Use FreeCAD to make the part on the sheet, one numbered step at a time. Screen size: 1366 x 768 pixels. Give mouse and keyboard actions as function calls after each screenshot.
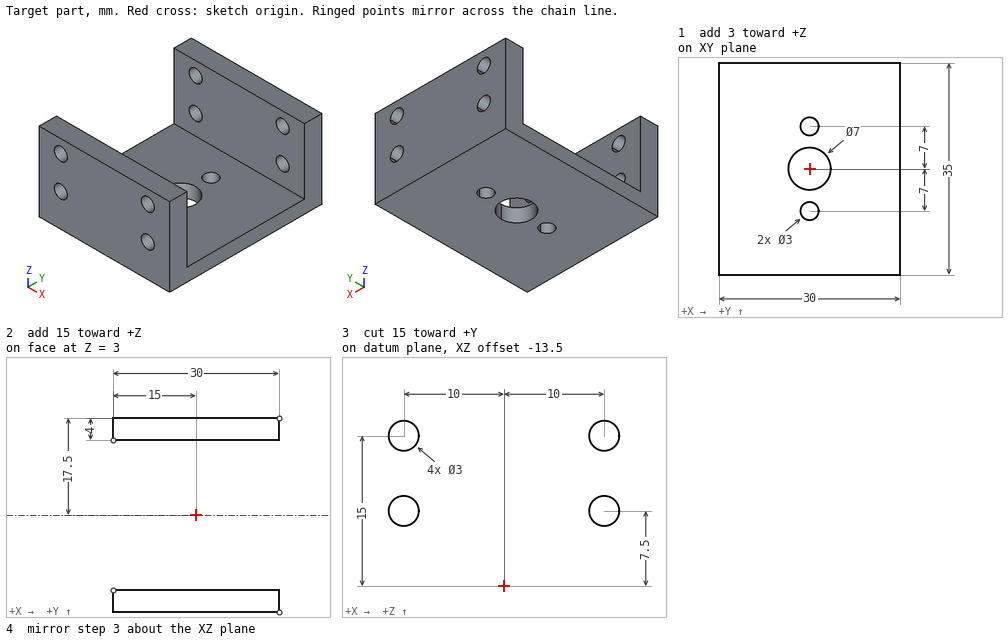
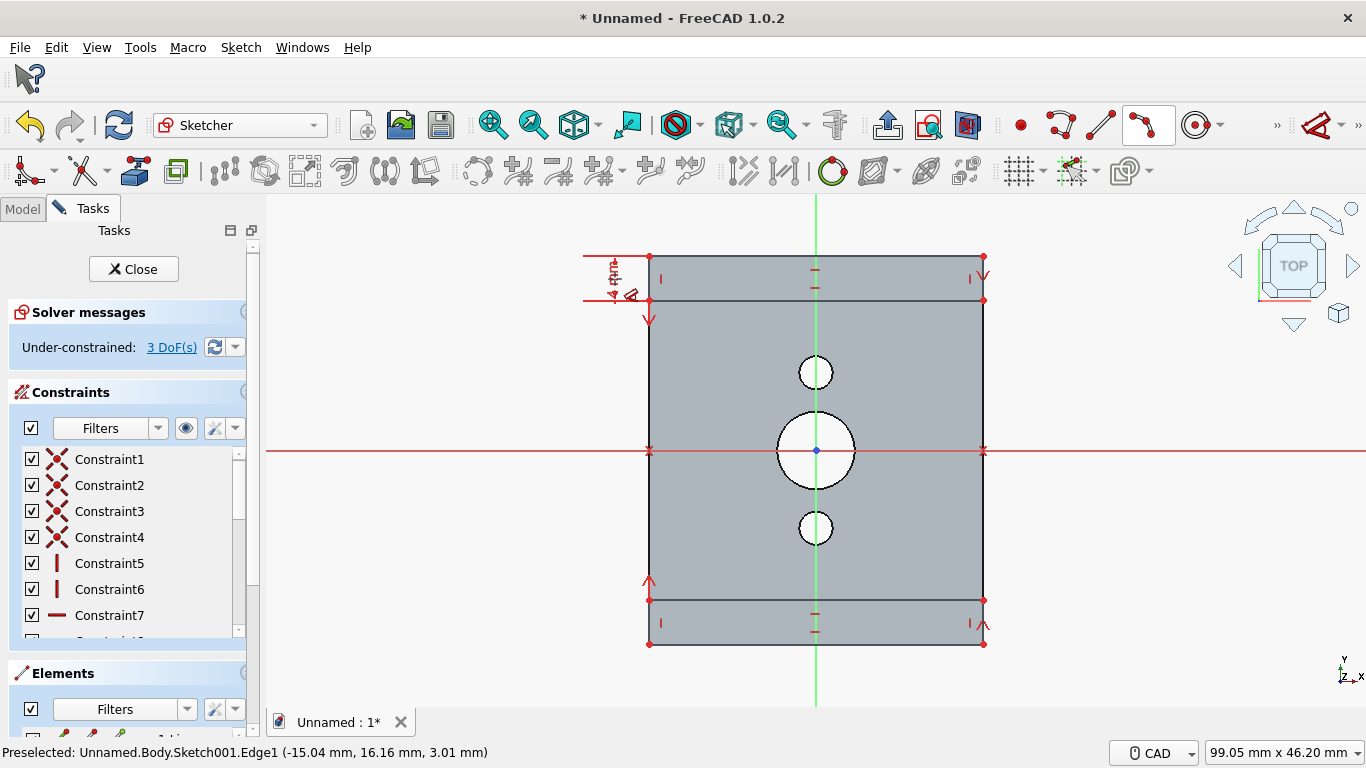
click(749, 301)
click(739, 335)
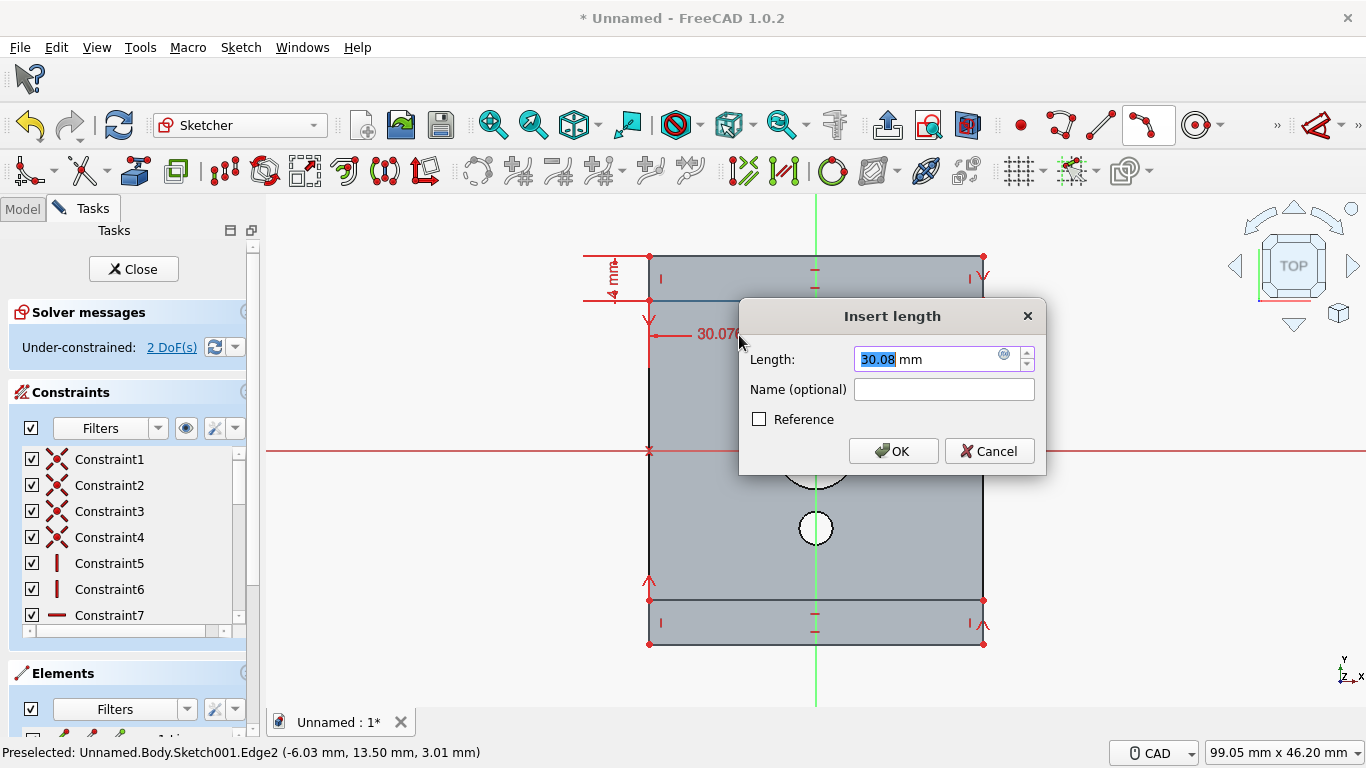
text(30)
key(Return)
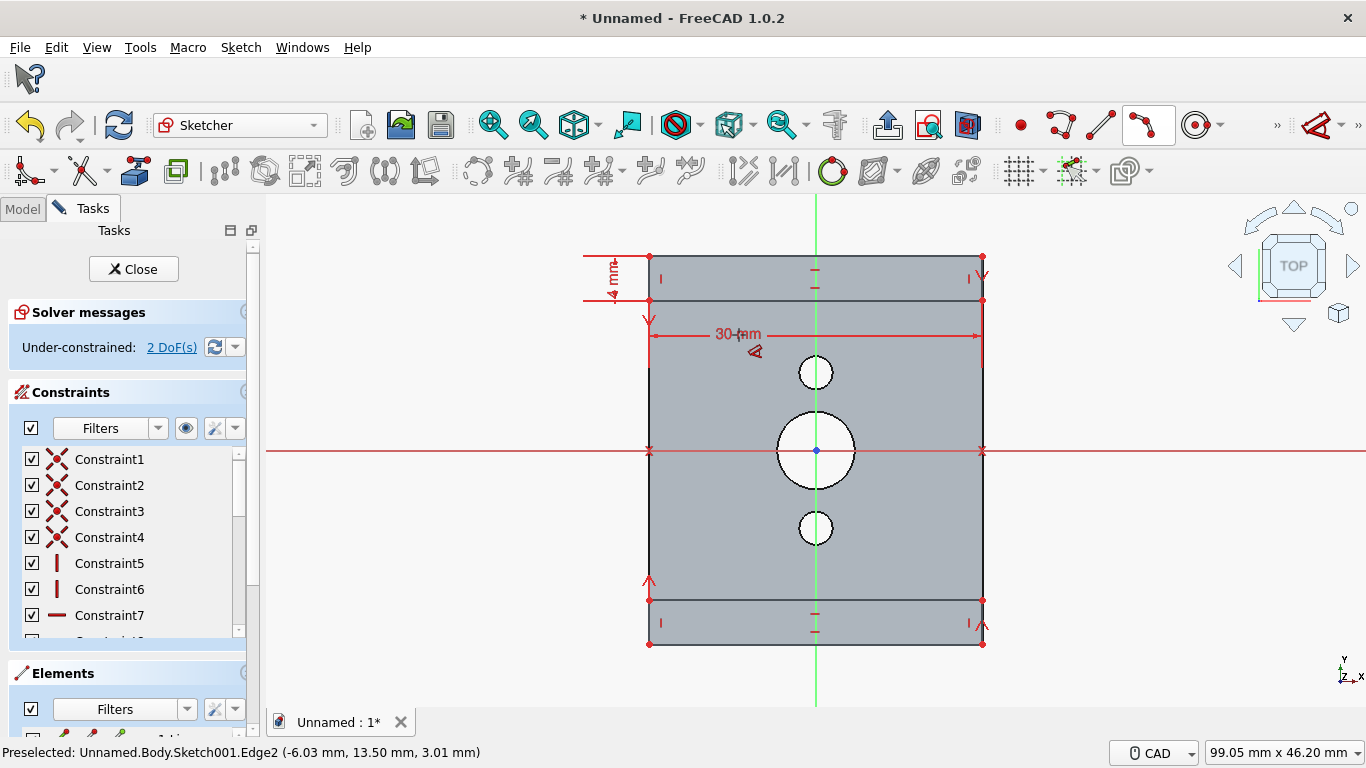
click(649, 256)
click(733, 222)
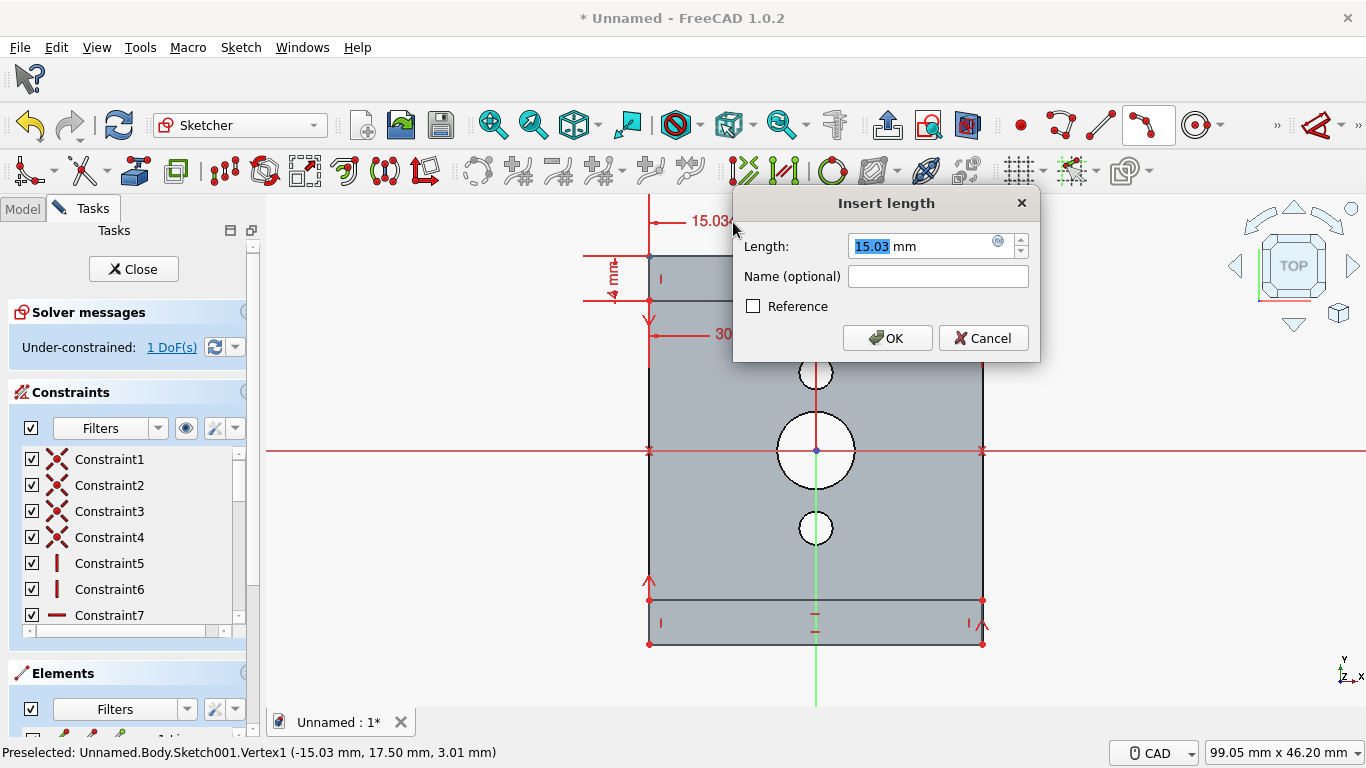
text(15)
key(Return)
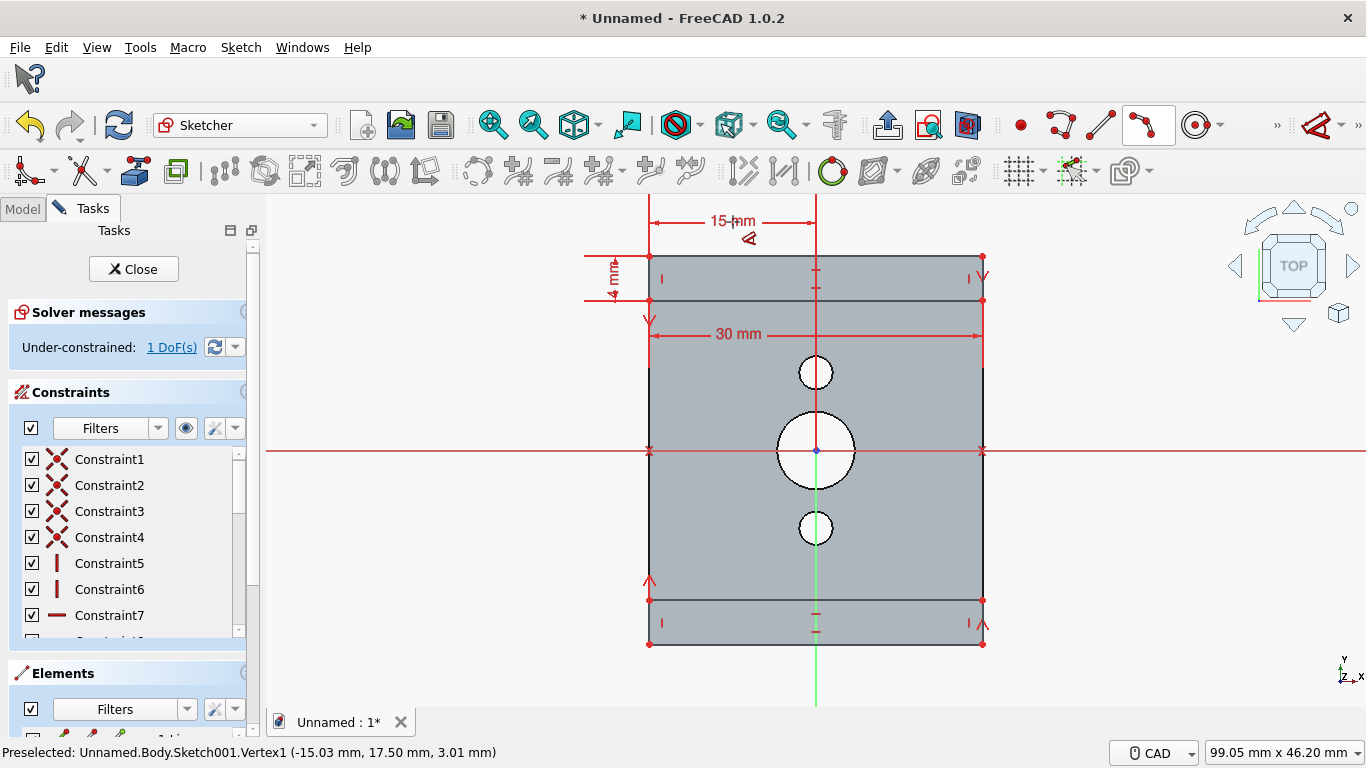
click(649, 256)
click(615, 353)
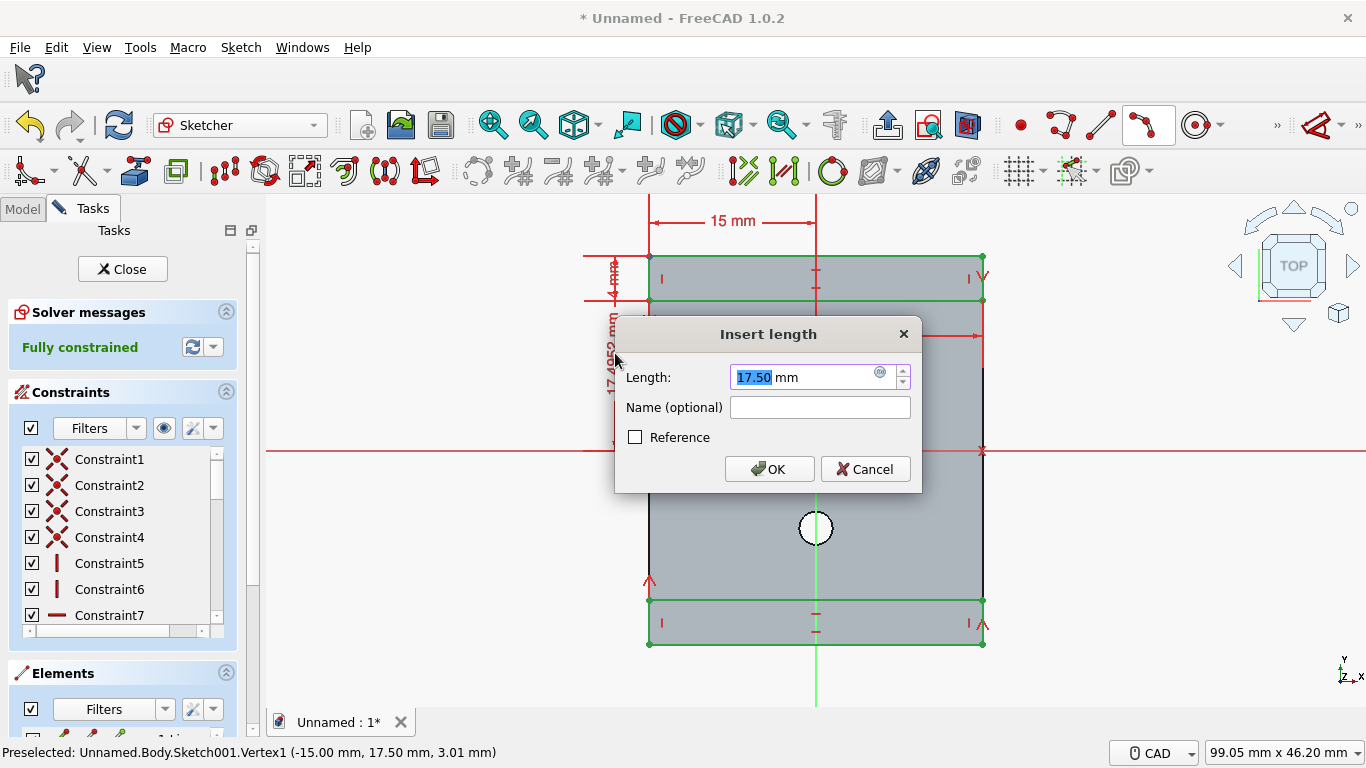
text(17.5)
key(Return)
key(Escape)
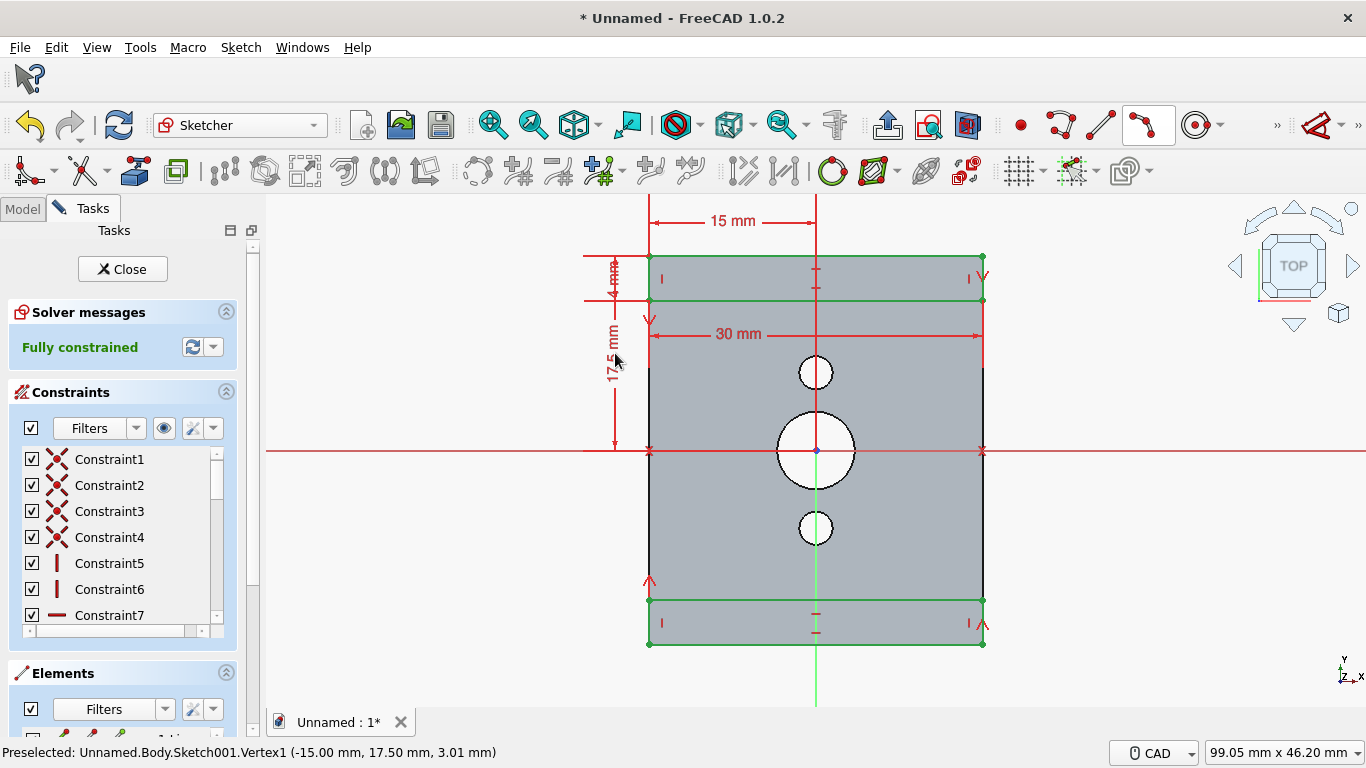
click(123, 269)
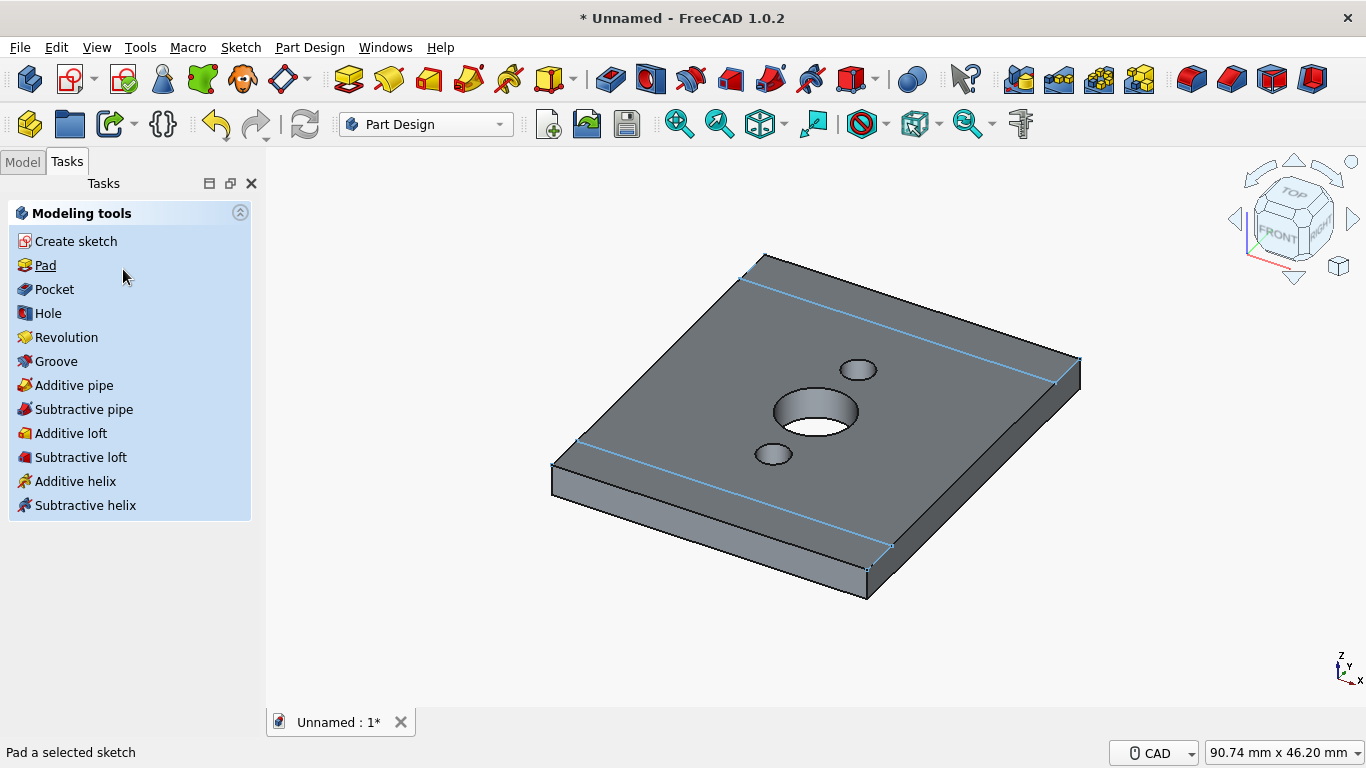
click(350, 80)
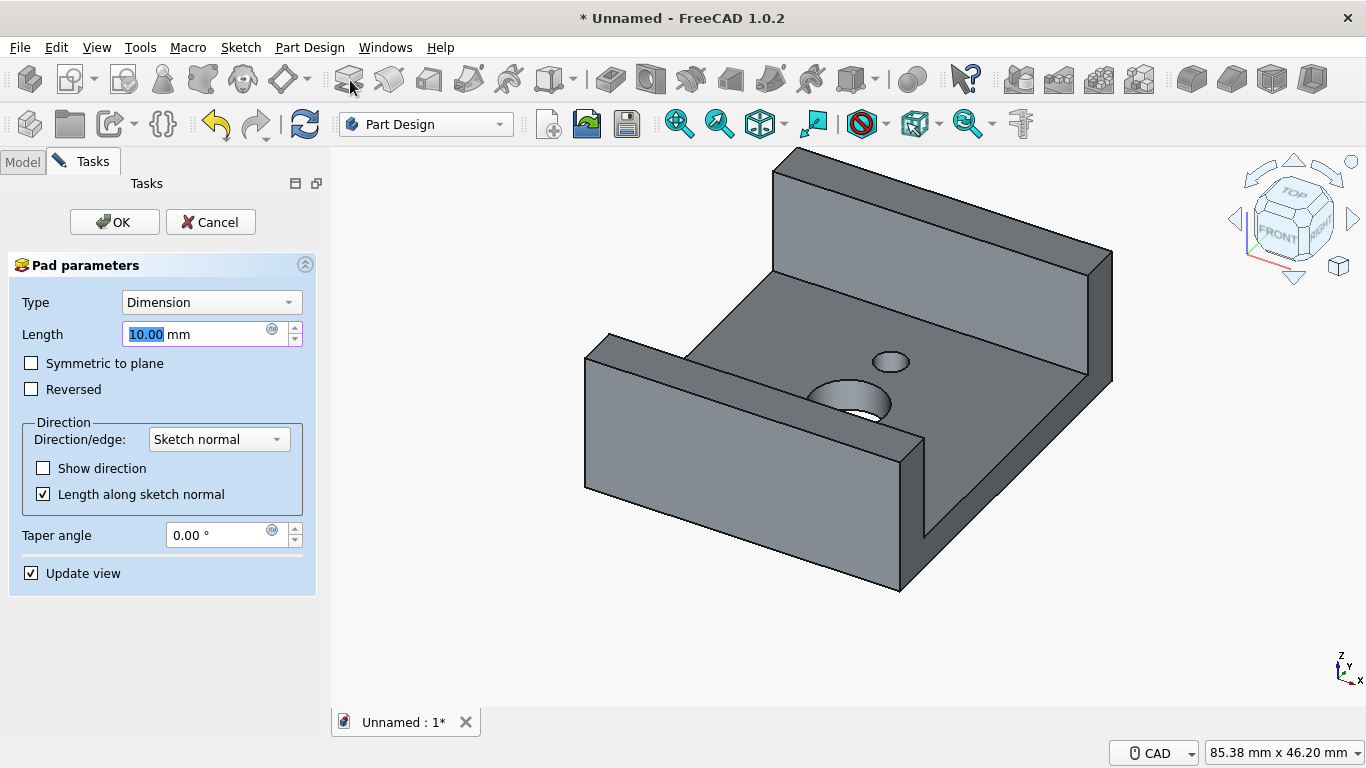
text(15)
key(Tab)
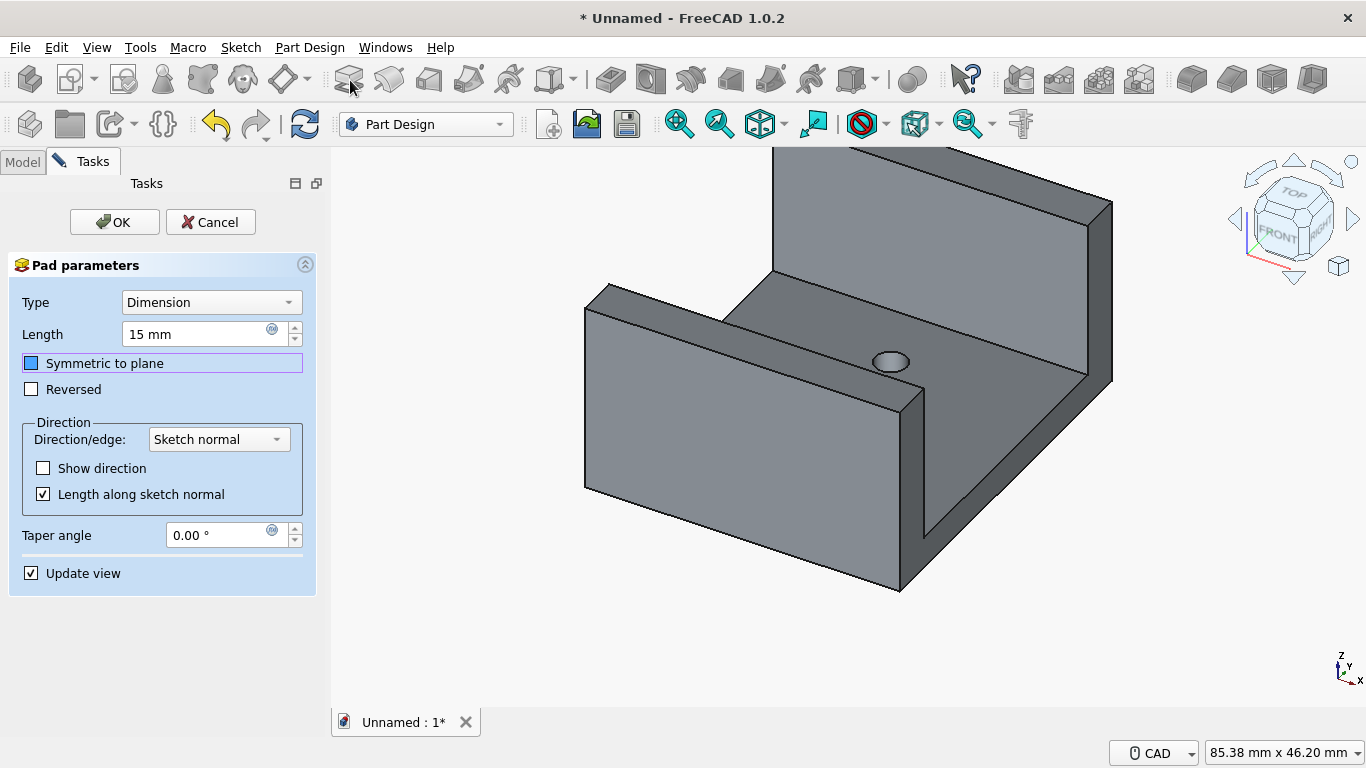
click(115, 222)